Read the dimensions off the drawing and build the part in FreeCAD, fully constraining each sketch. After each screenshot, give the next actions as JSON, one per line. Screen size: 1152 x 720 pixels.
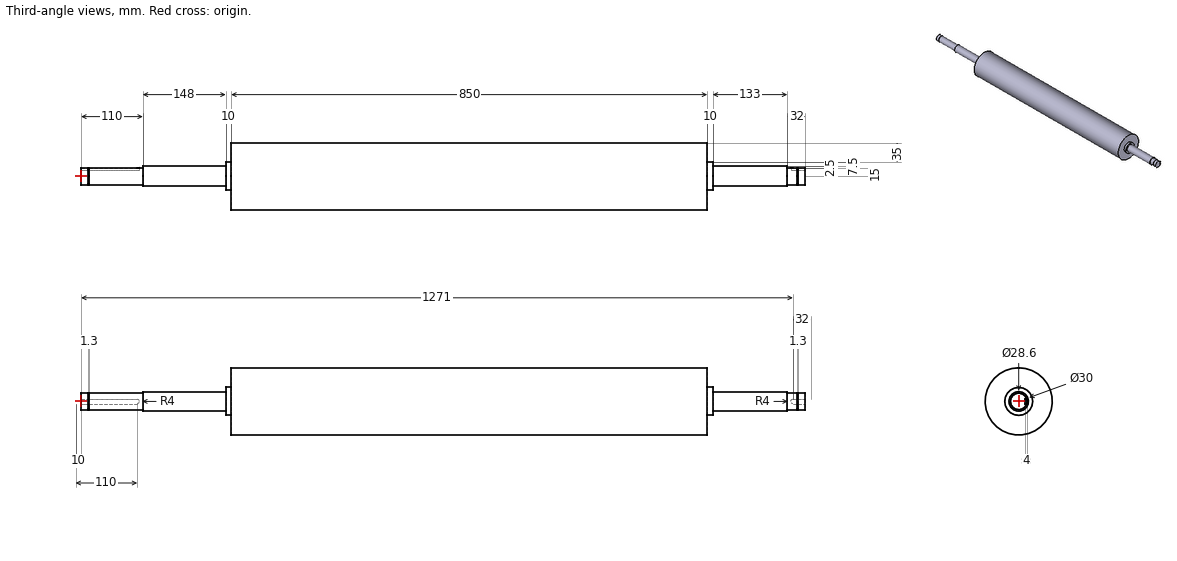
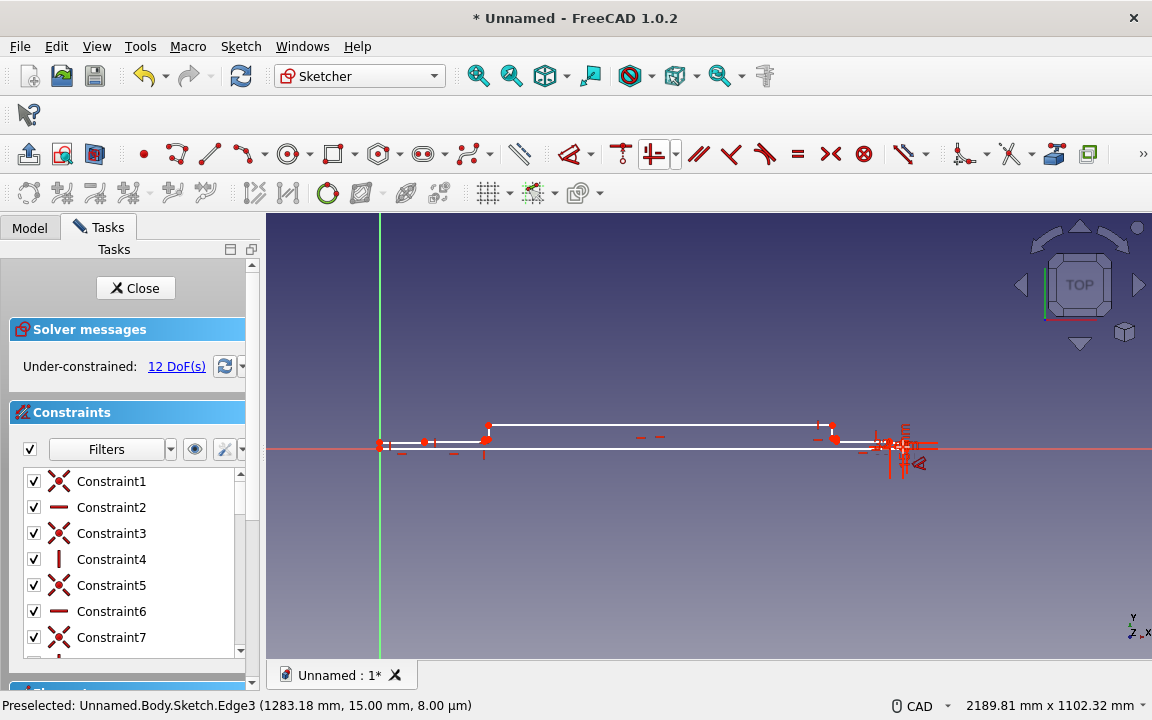
{"action": "scroll", "coordinate": [835, 439], "scroll_direction": "up", "scroll_amount": 13}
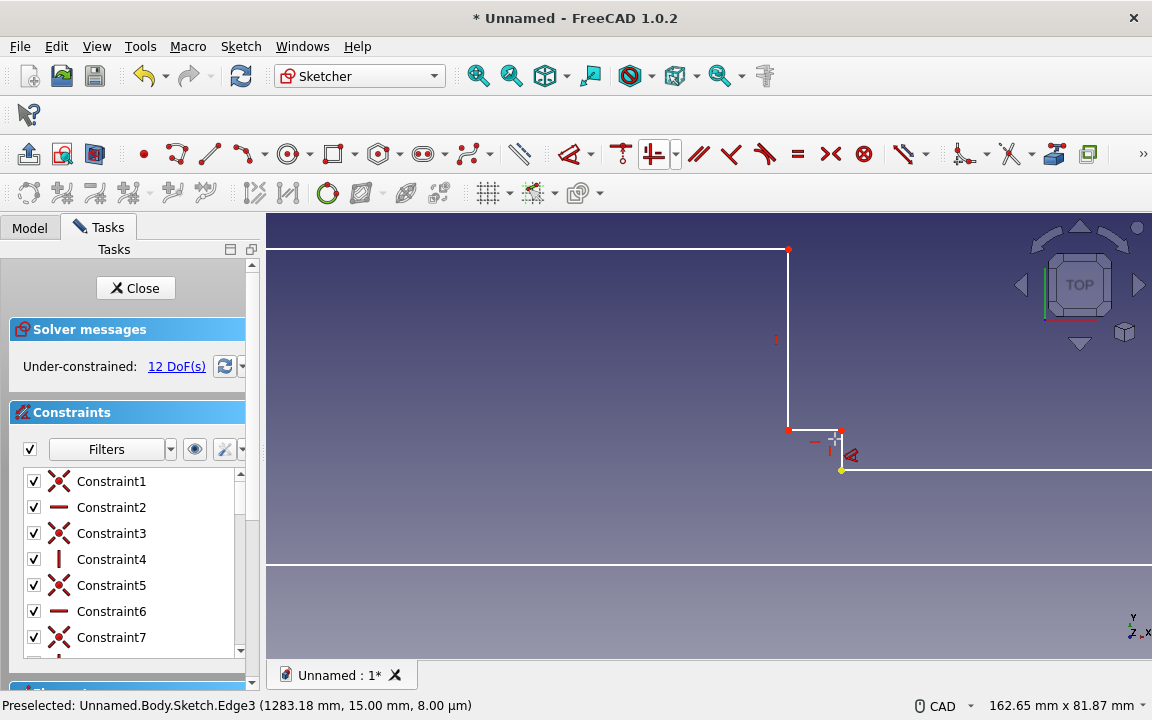
{"action": "left_click", "coordinate": [826, 430]}
{"action": "left_click", "coordinate": [815, 464]}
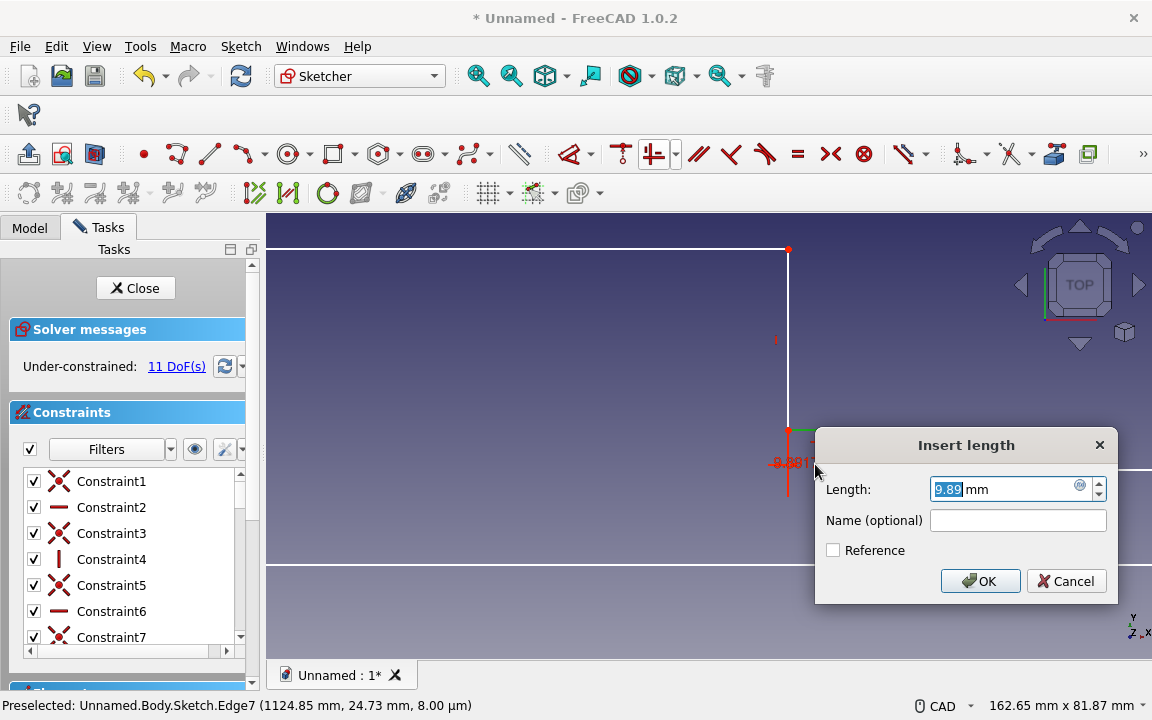
{"action": "type", "text": "10"}
{"action": "key", "text": "Return"}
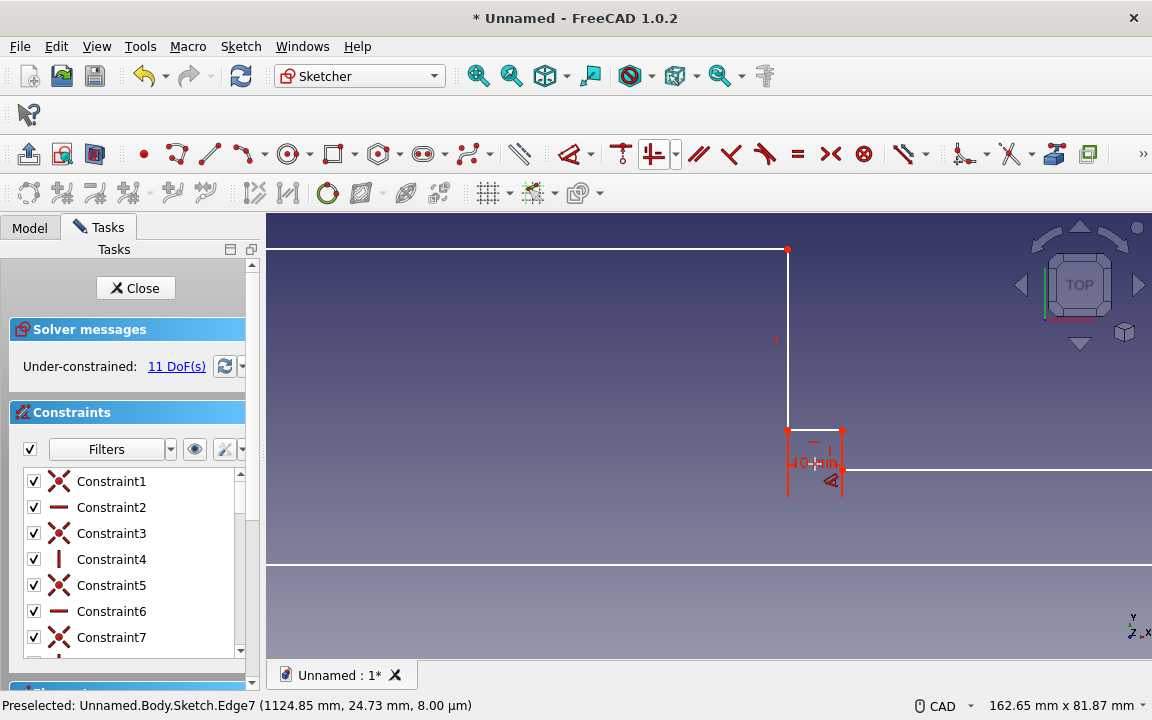
{"action": "scroll", "coordinate": [835, 439], "scroll_direction": "down", "scroll_amount": 13}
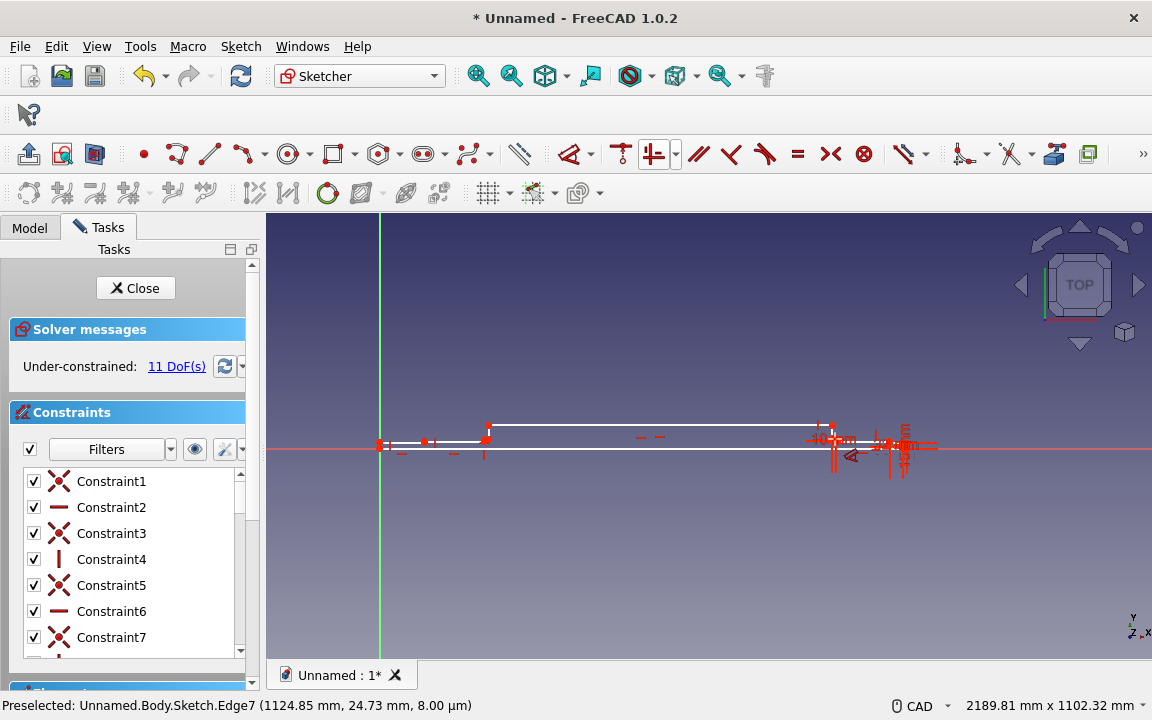
{"action": "scroll", "coordinate": [832, 435], "scroll_direction": "up", "scroll_amount": 7}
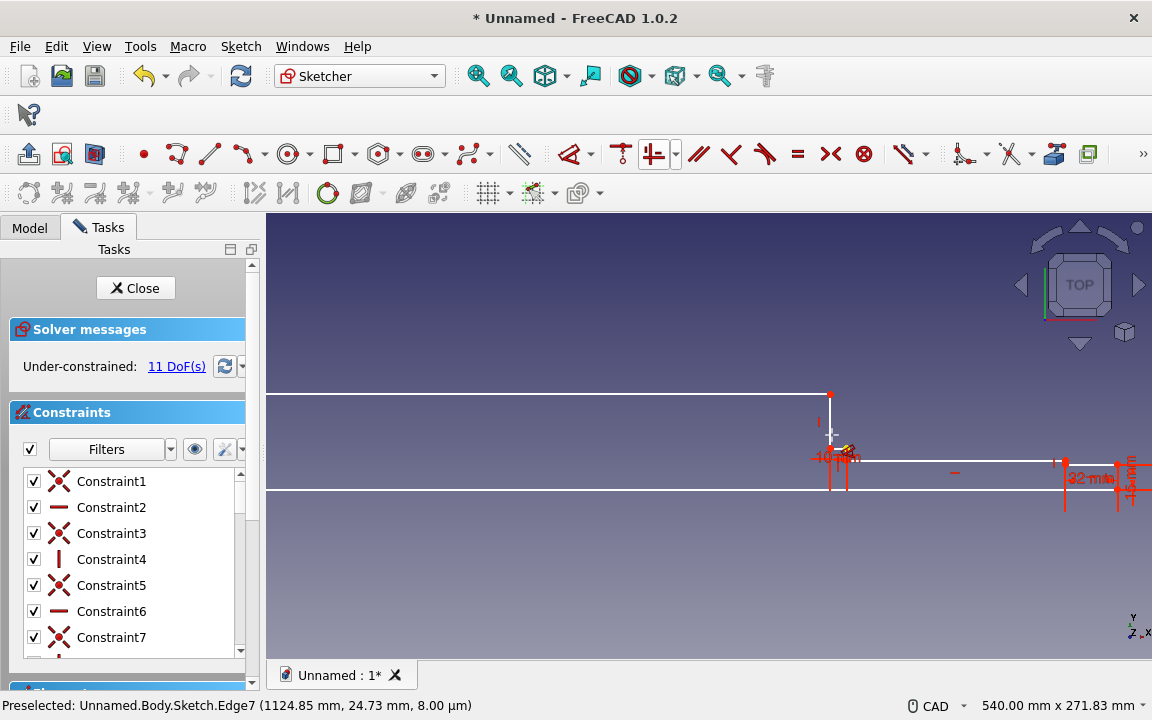
{"action": "left_click", "coordinate": [830, 433]}
{"action": "left_click", "coordinate": [864, 422]}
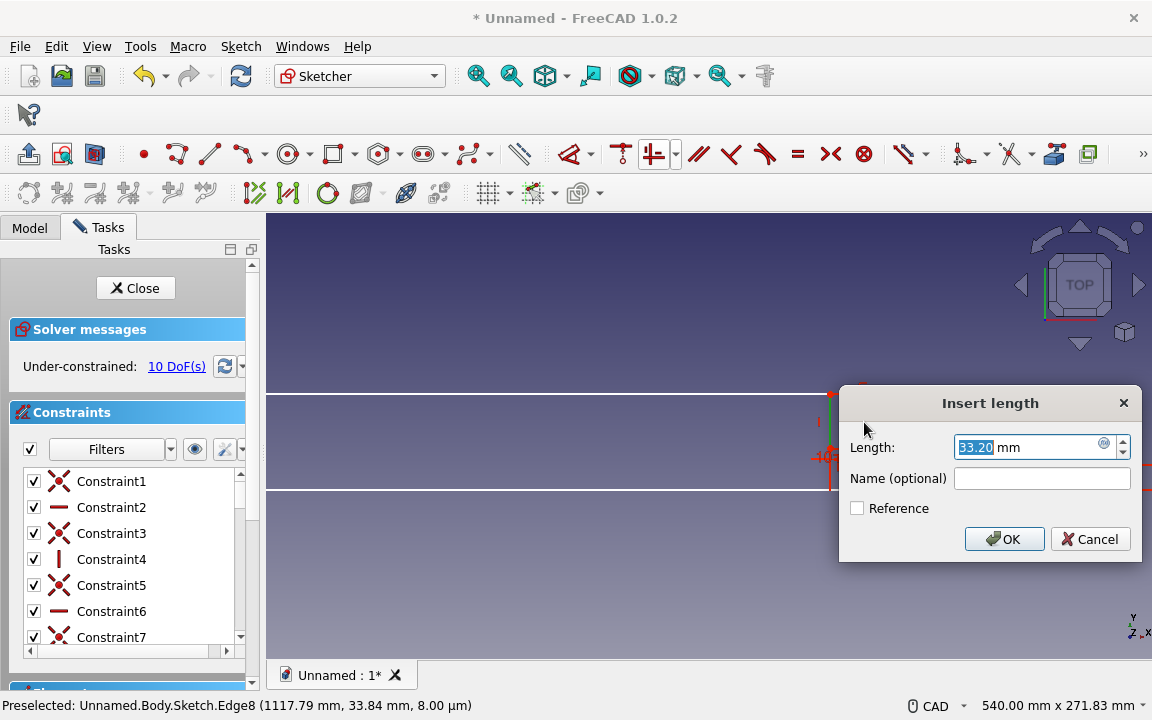
{"action": "type", "text": "35"}
{"action": "key", "text": "Return"}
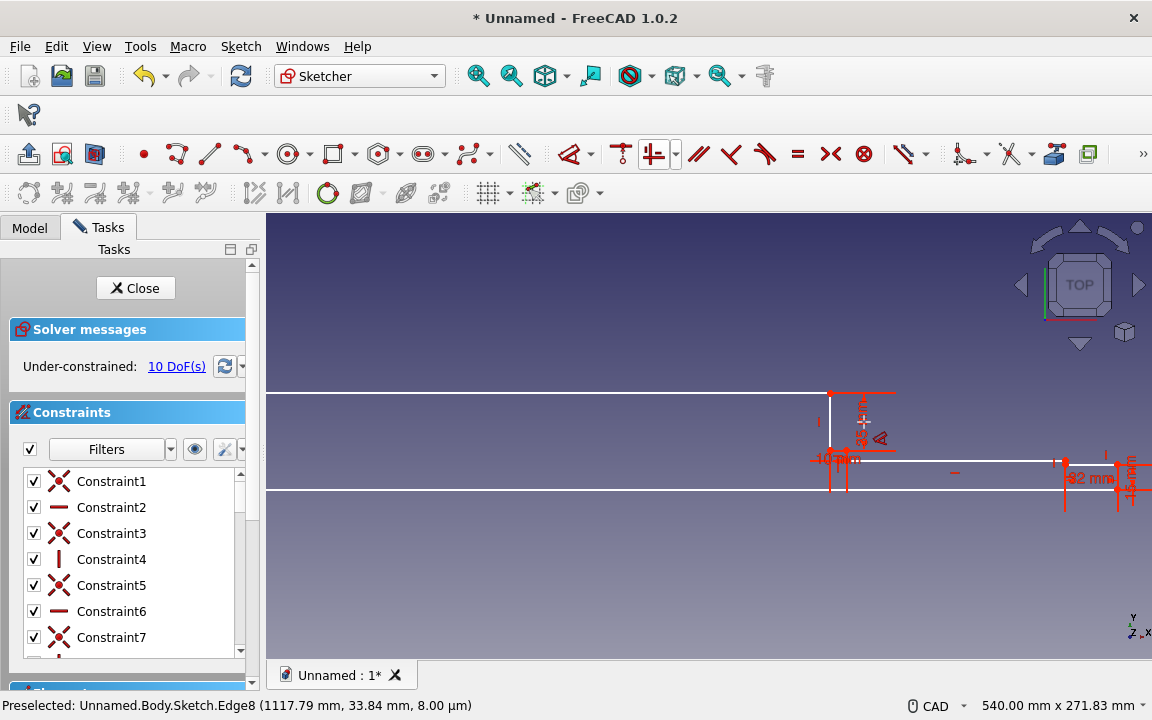
{"action": "scroll", "coordinate": [831, 435], "scroll_direction": "down", "scroll_amount": 7}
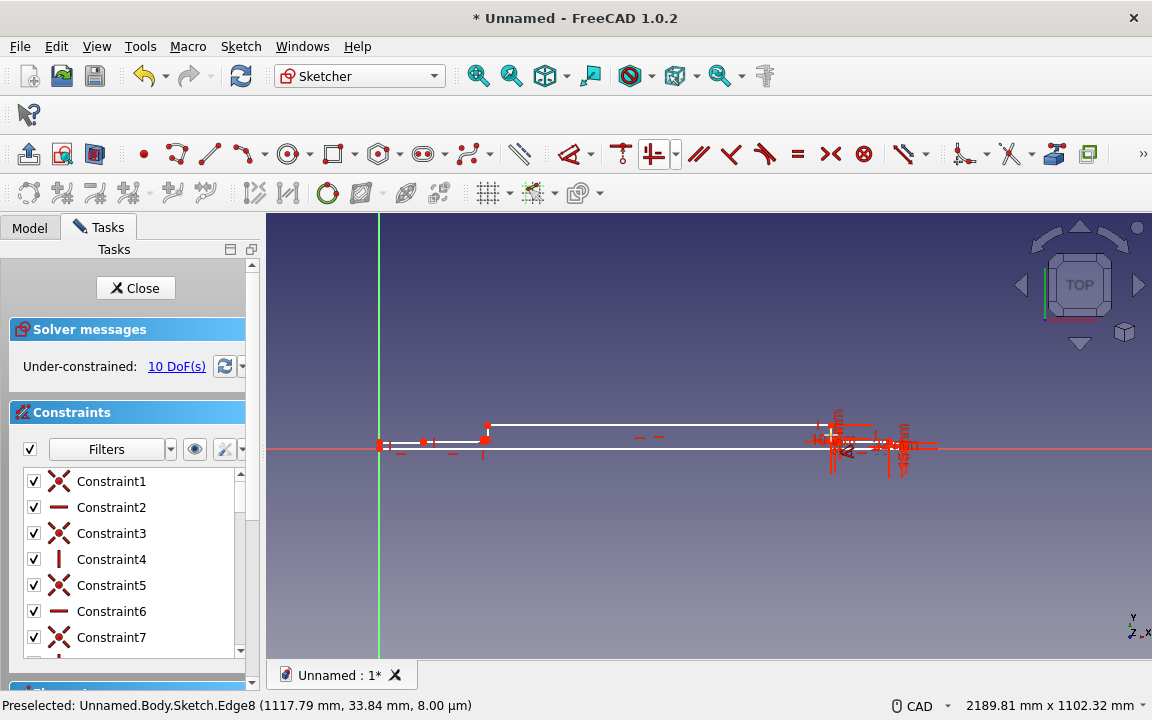
{"action": "scroll", "coordinate": [488, 429], "scroll_direction": "up", "scroll_amount": 6}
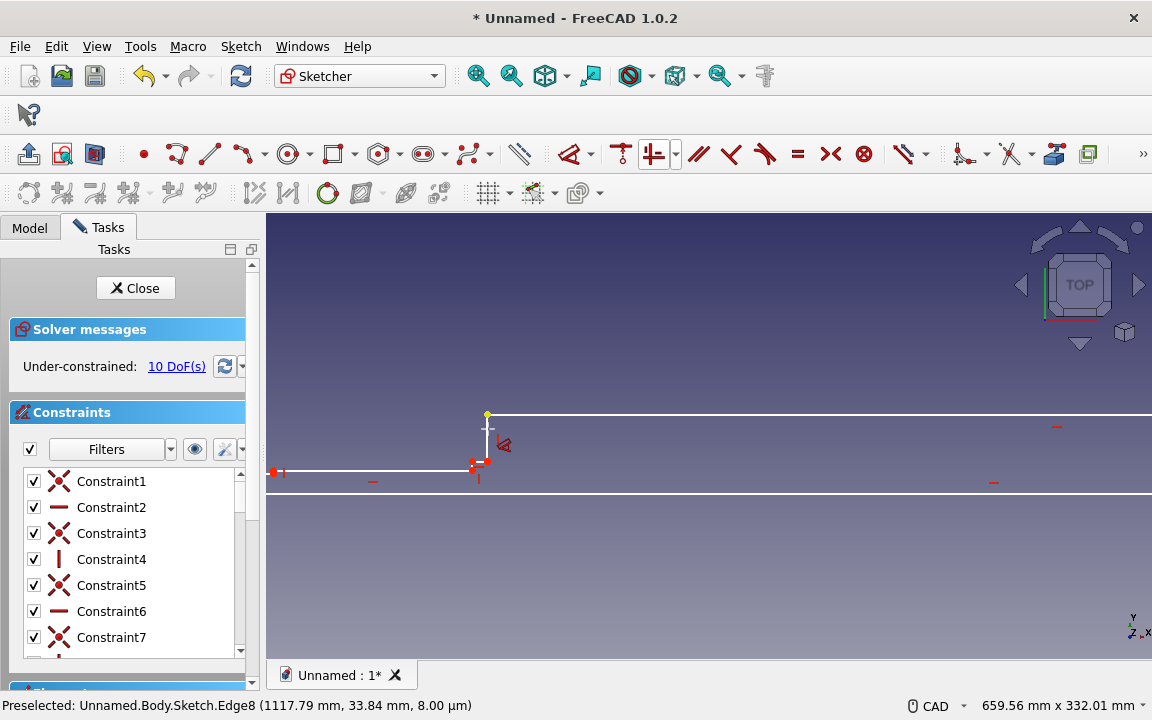
{"action": "left_click", "coordinate": [487, 429]}
{"action": "left_click", "coordinate": [453, 438]}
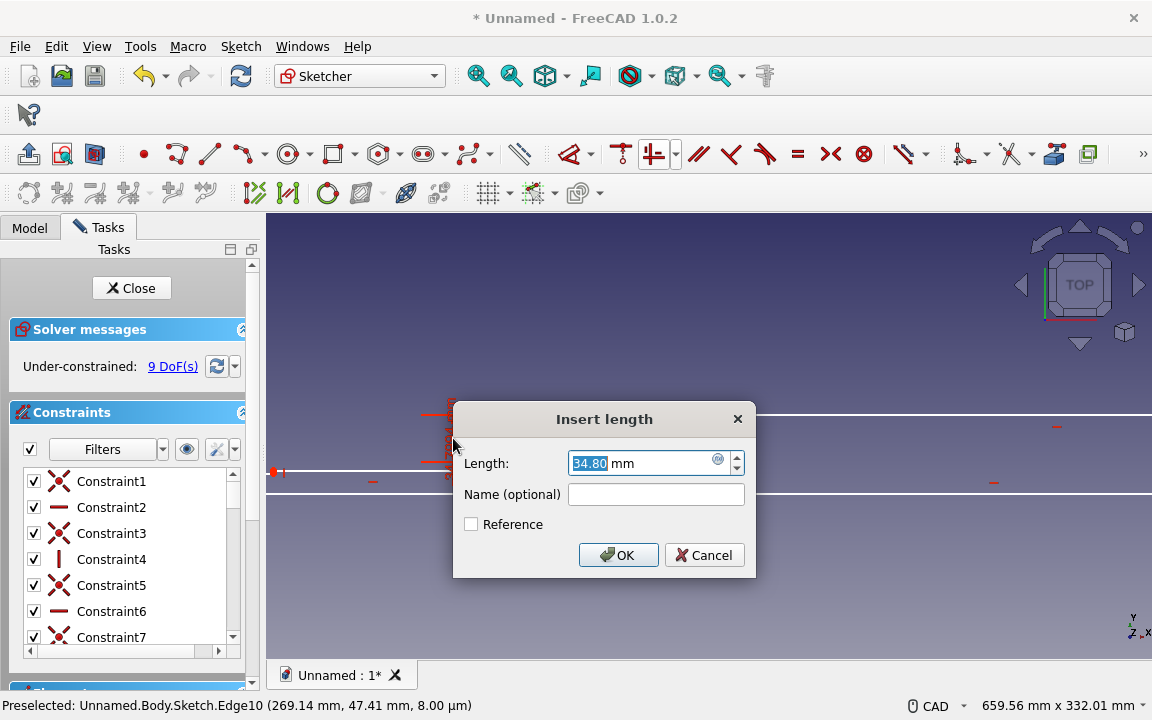
{"action": "type", "text": "35"}
{"action": "key", "text": "Return"}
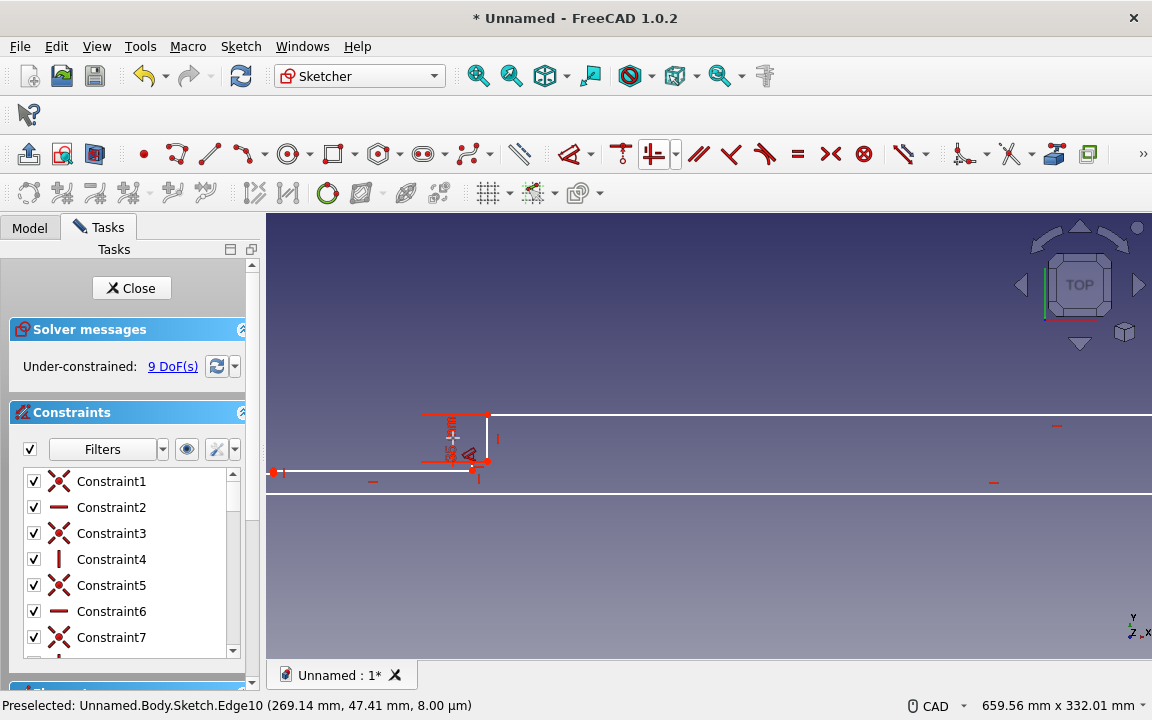
{"action": "scroll", "coordinate": [480, 462], "scroll_direction": "up", "scroll_amount": 6}